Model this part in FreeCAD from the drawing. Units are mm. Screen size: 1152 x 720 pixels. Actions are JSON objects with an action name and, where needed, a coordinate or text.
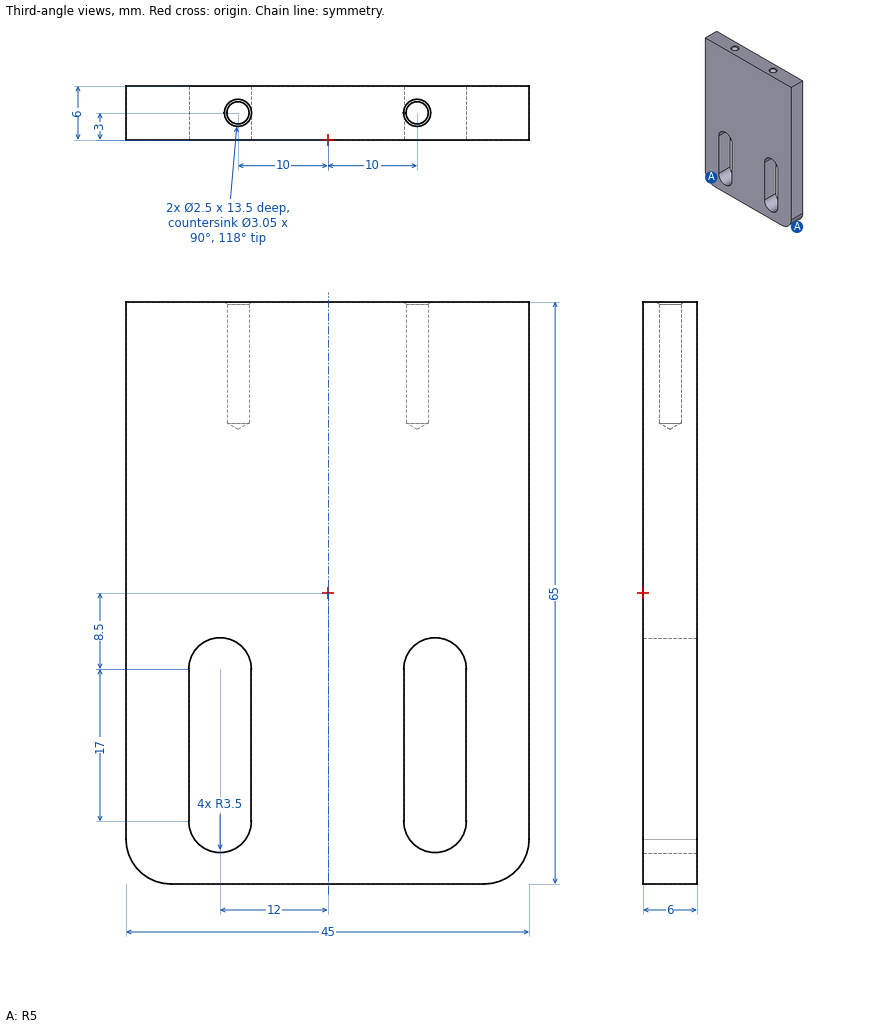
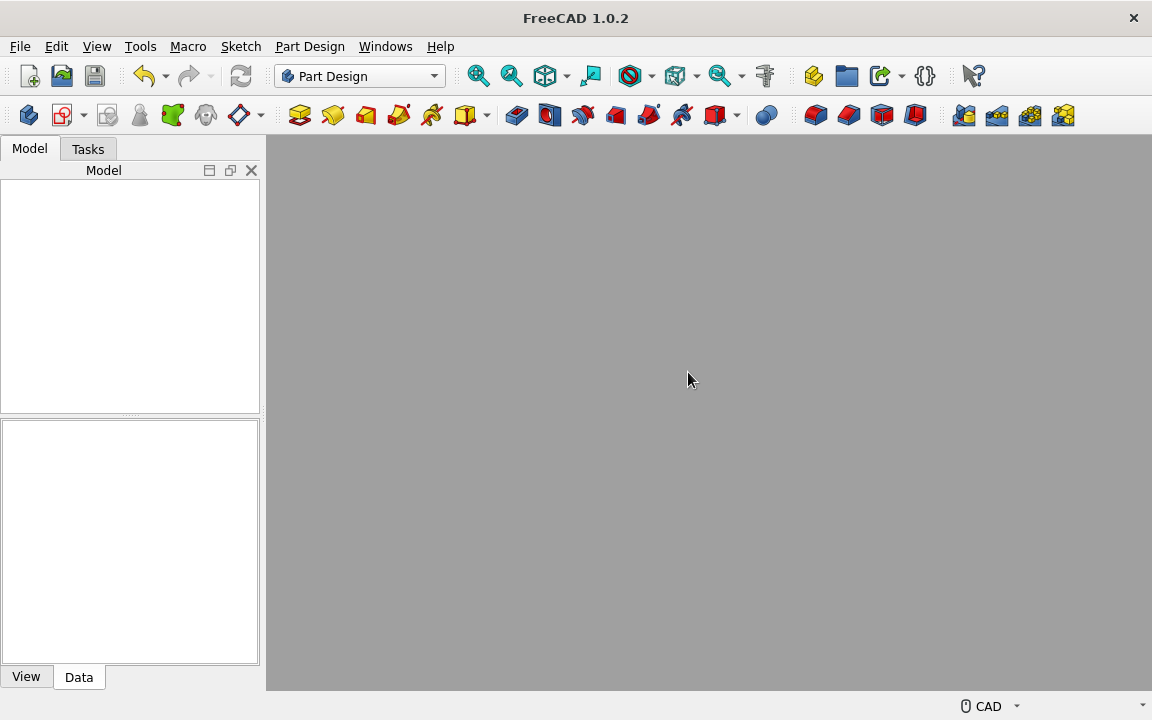
{"action": "left_click", "coordinate": [29, 76]}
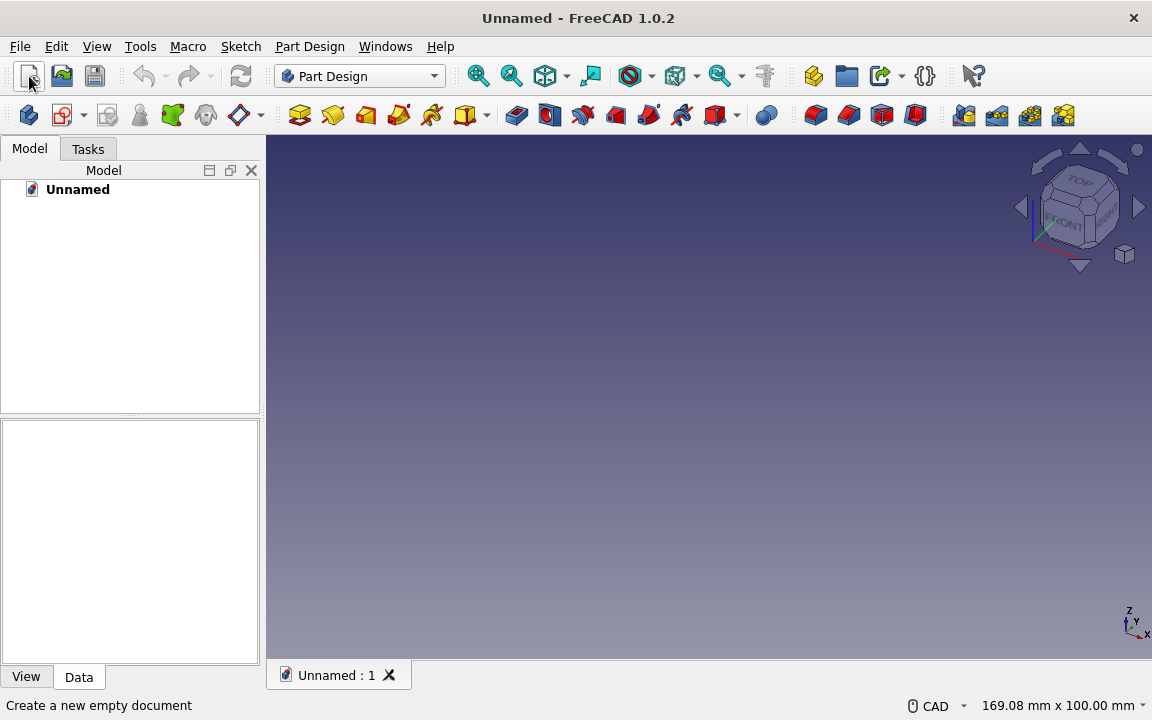
{"action": "left_click", "coordinate": [62, 116]}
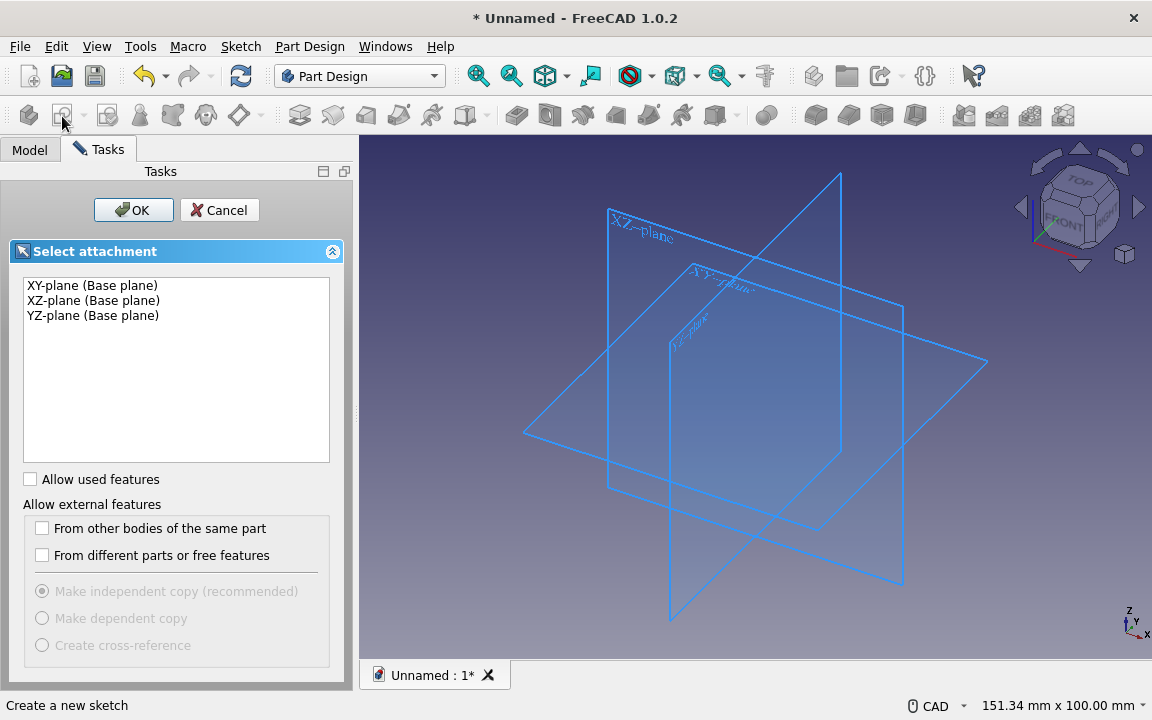
{"action": "left_click", "coordinate": [84, 300]}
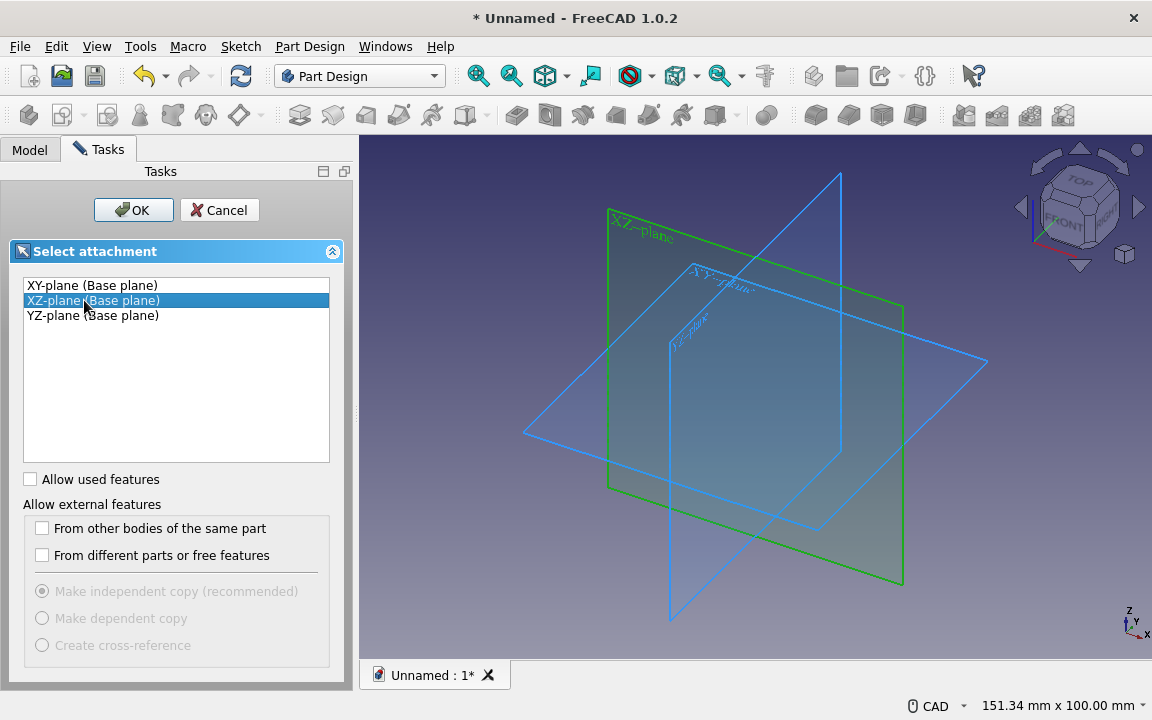
{"action": "left_click", "coordinate": [134, 210]}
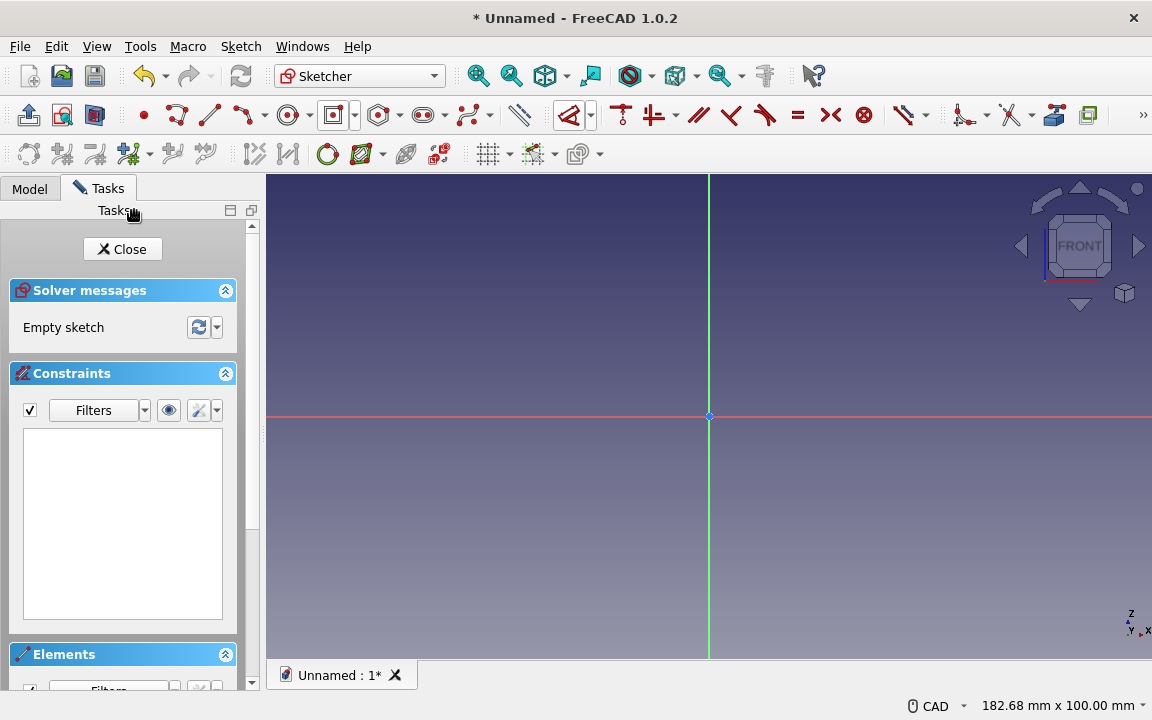
{"action": "key", "text": "g v"}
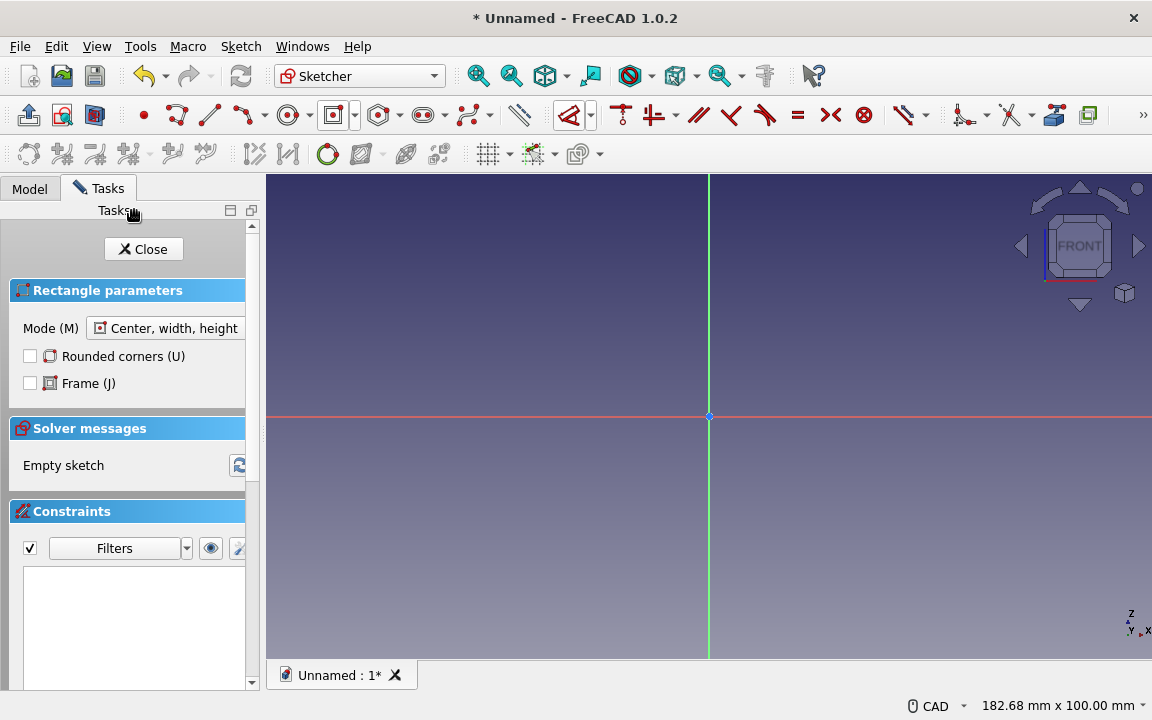
{"action": "left_click", "coordinate": [709, 416]}
{"action": "mouse_move", "coordinate": [818, 259]}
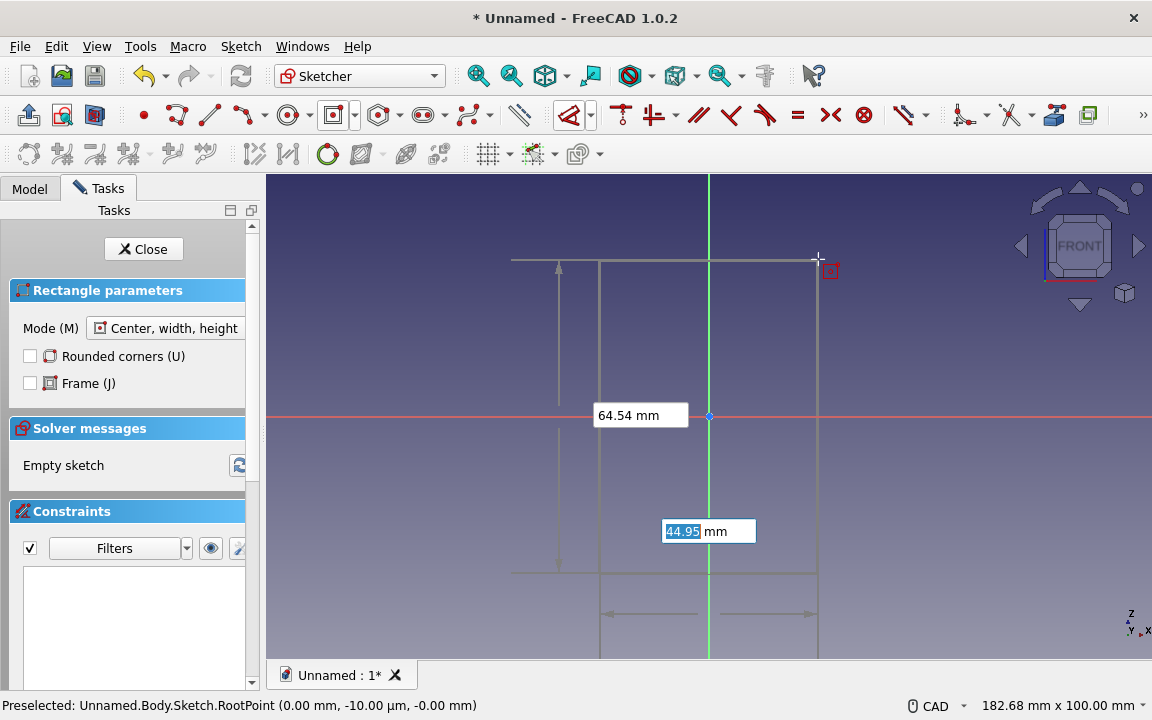
{"action": "type", "text": "45"}
{"action": "key", "text": "Tab"}
{"action": "type", "text": "65"}
{"action": "key", "text": "Return"}
{"action": "key", "text": "Escape"}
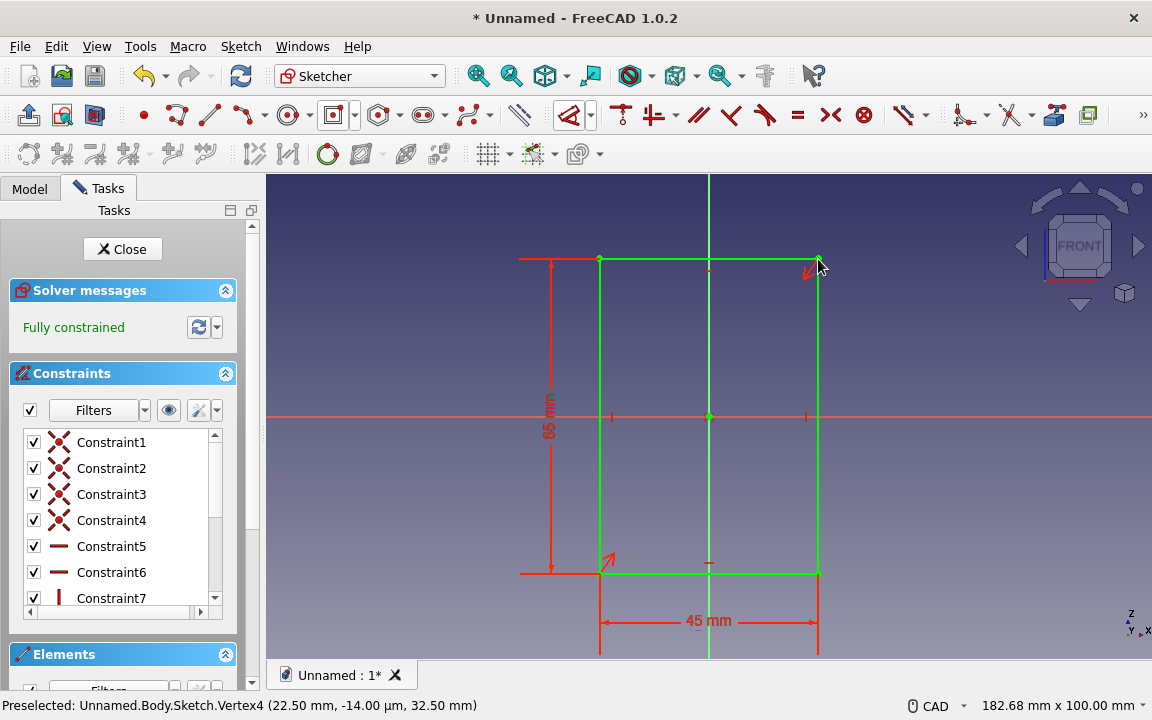
{"action": "left_click", "coordinate": [123, 249]}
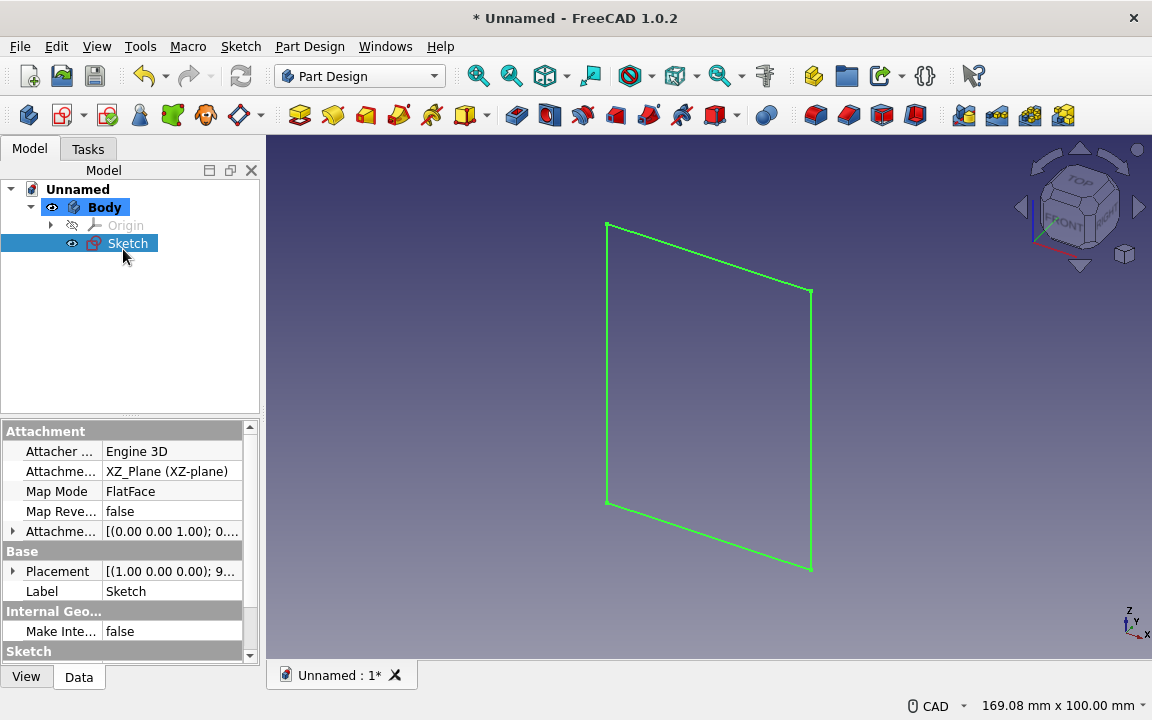
{"action": "left_click", "coordinate": [300, 116]}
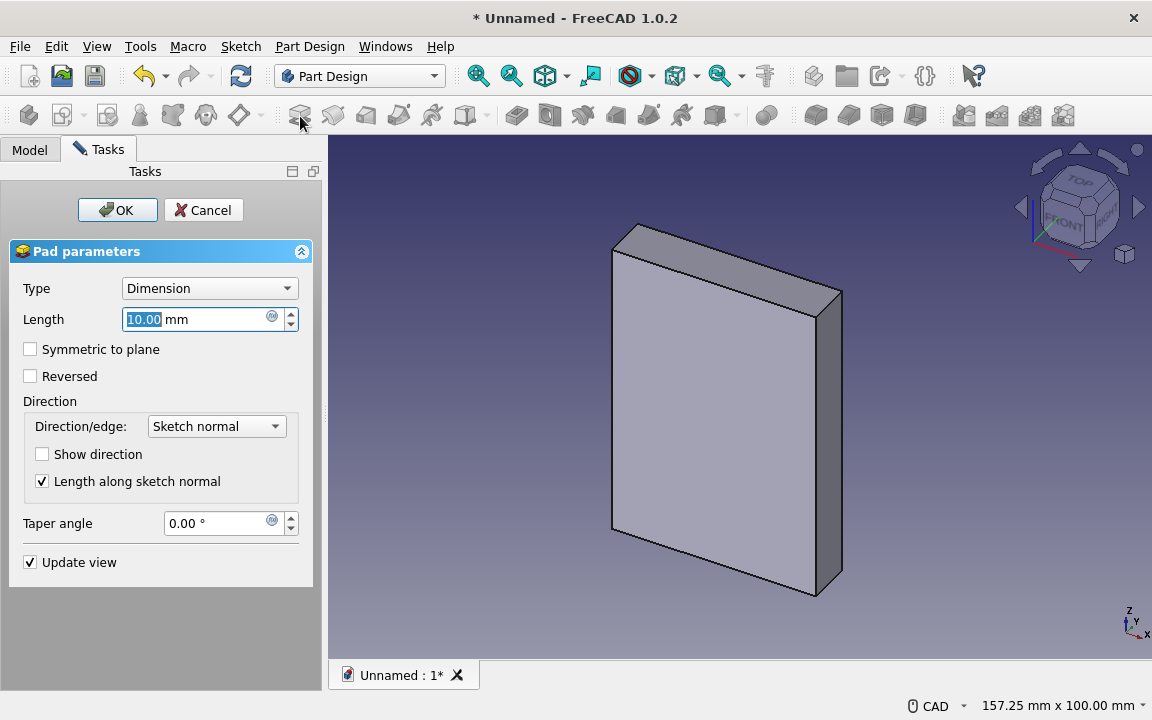
{"action": "type", "text": "6"}
{"action": "key", "text": "Tab"}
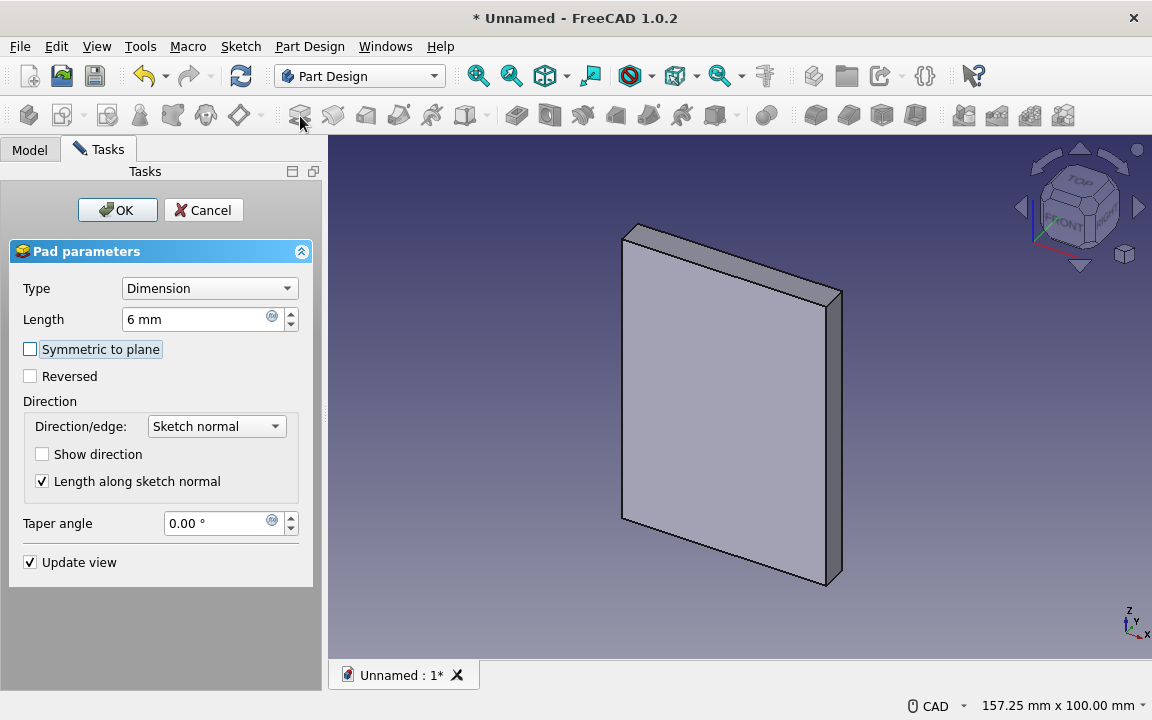
{"action": "left_click", "coordinate": [31, 376]}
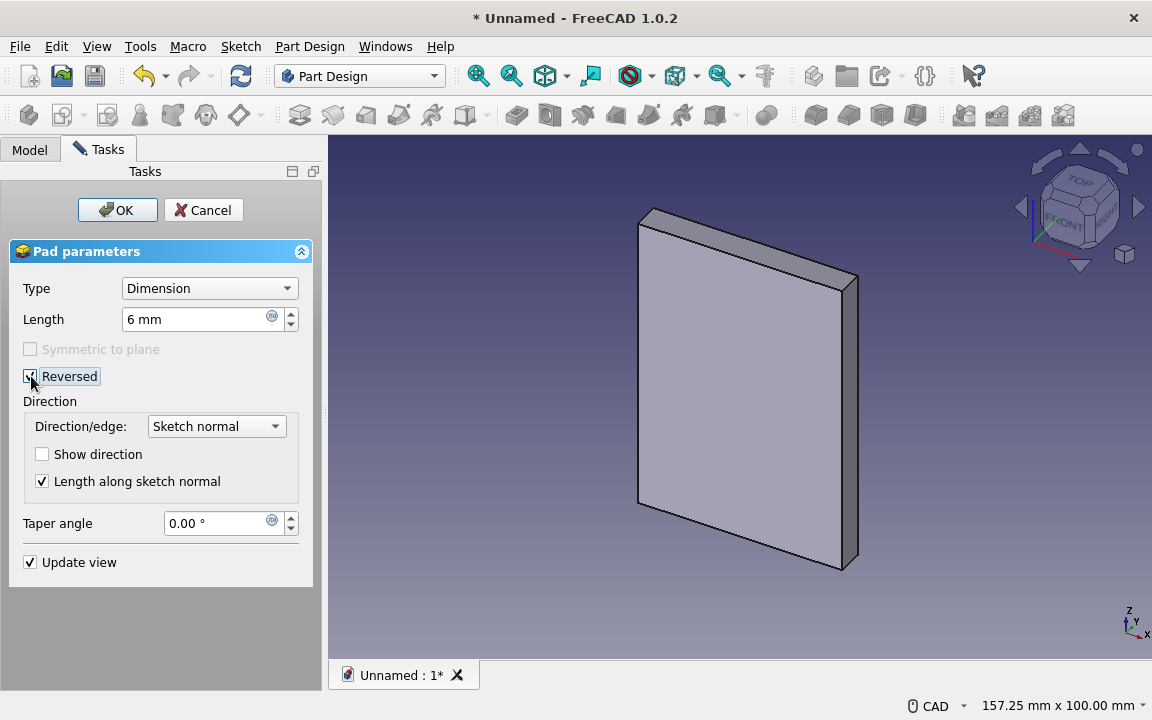
{"action": "left_click", "coordinate": [118, 210]}